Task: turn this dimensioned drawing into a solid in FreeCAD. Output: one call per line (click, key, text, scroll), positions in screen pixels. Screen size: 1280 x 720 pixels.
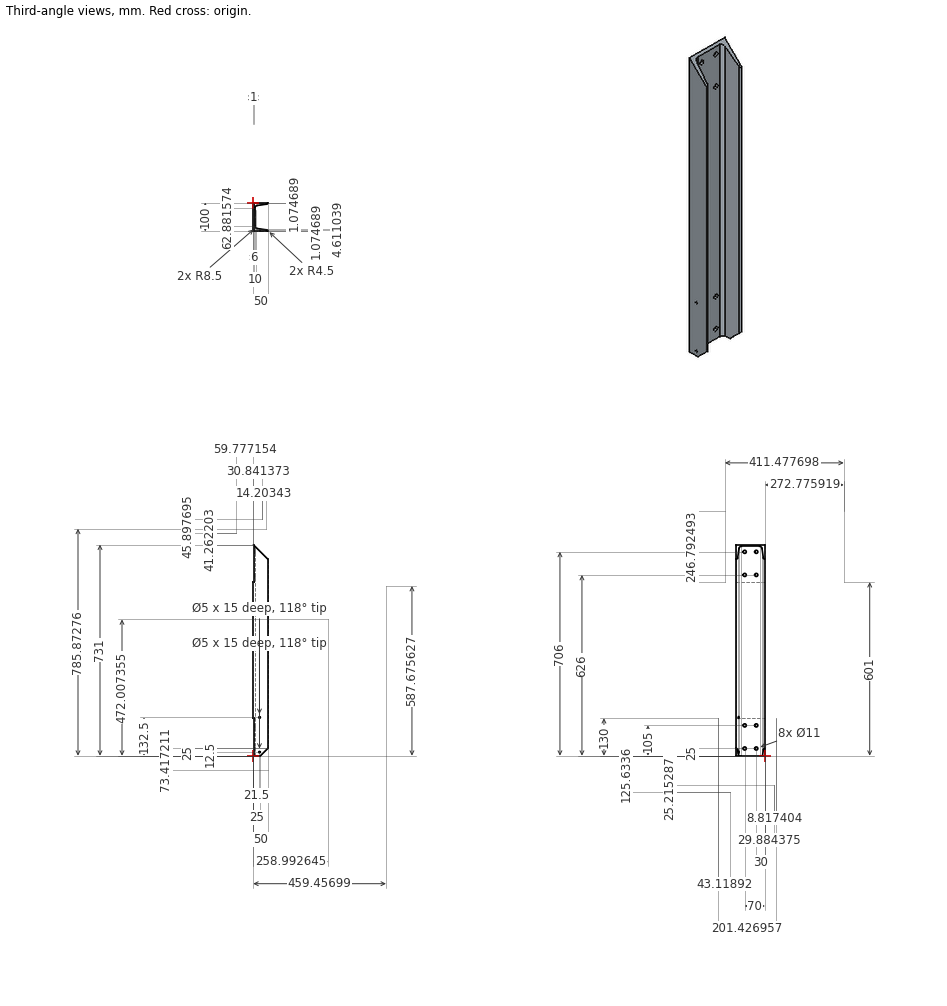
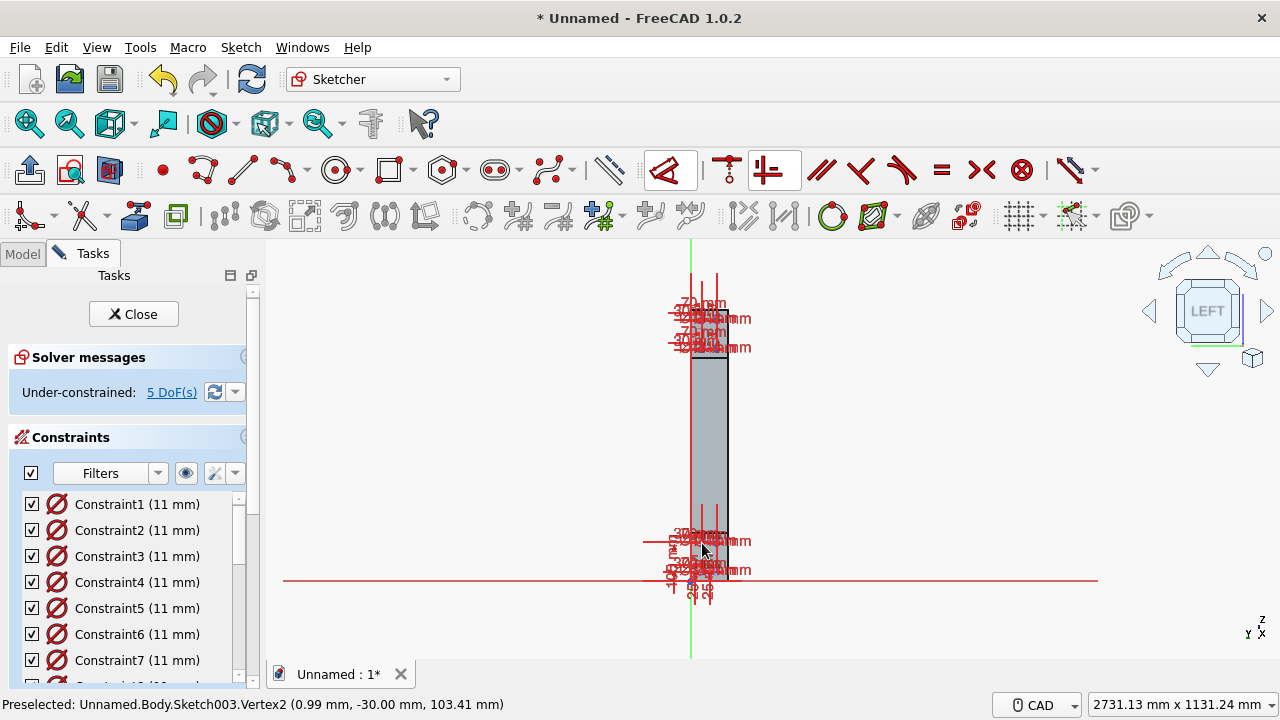
click(717, 543)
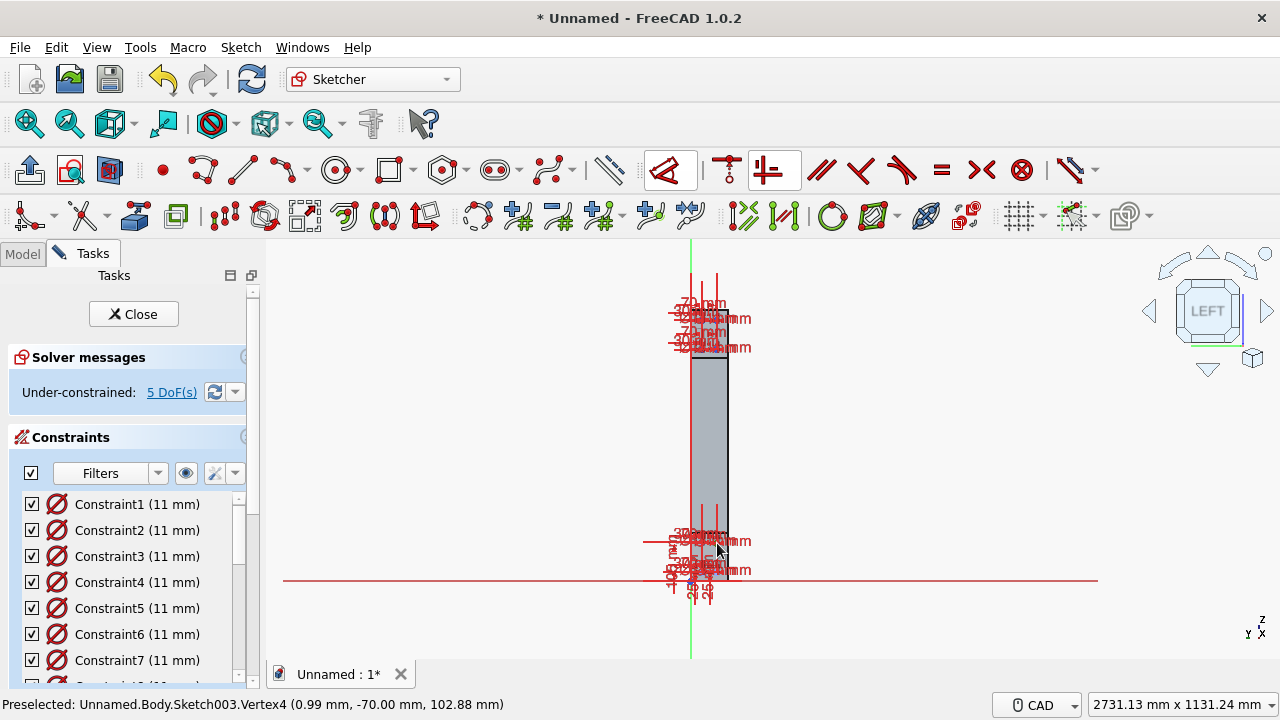
key(i)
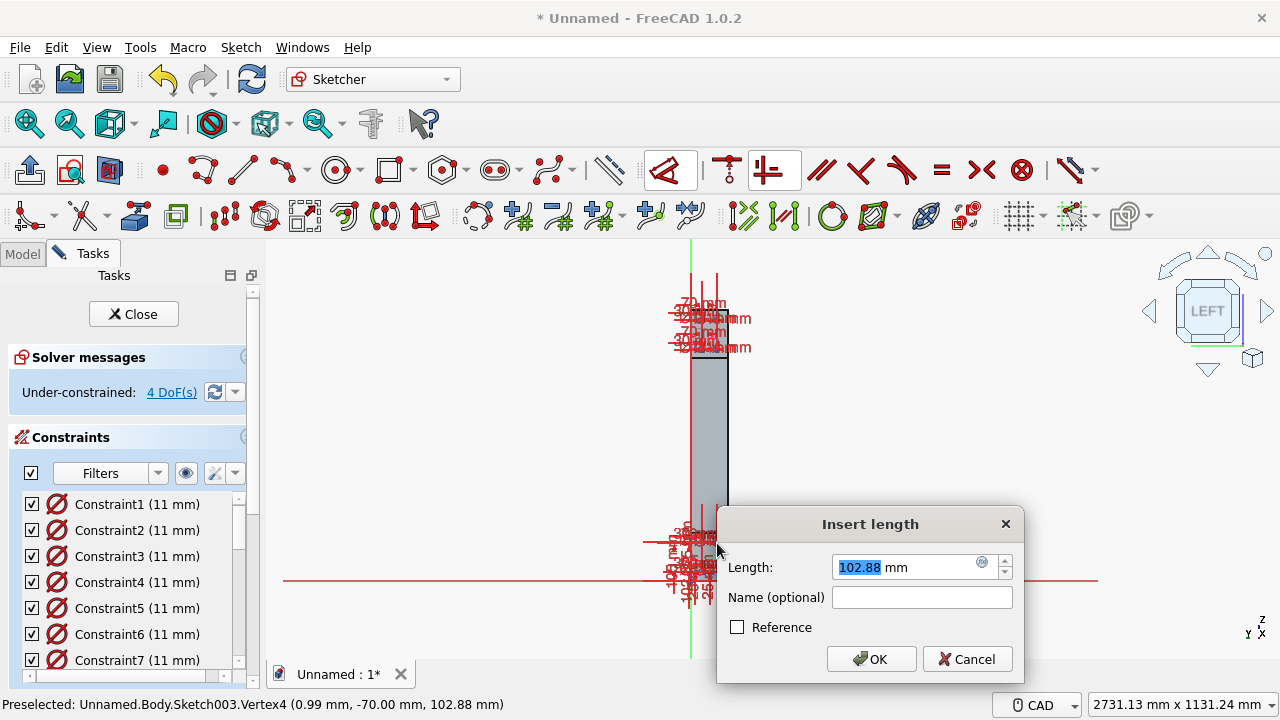
text(105)
key(Return)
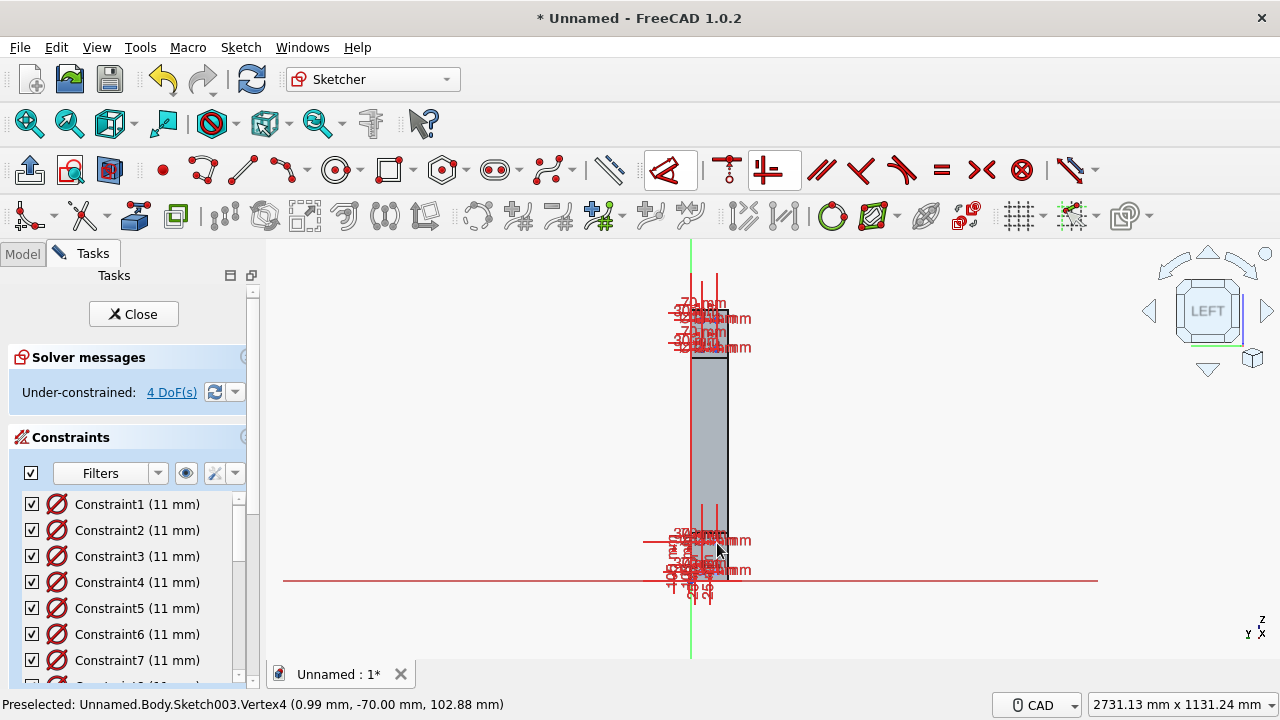
click(702, 350)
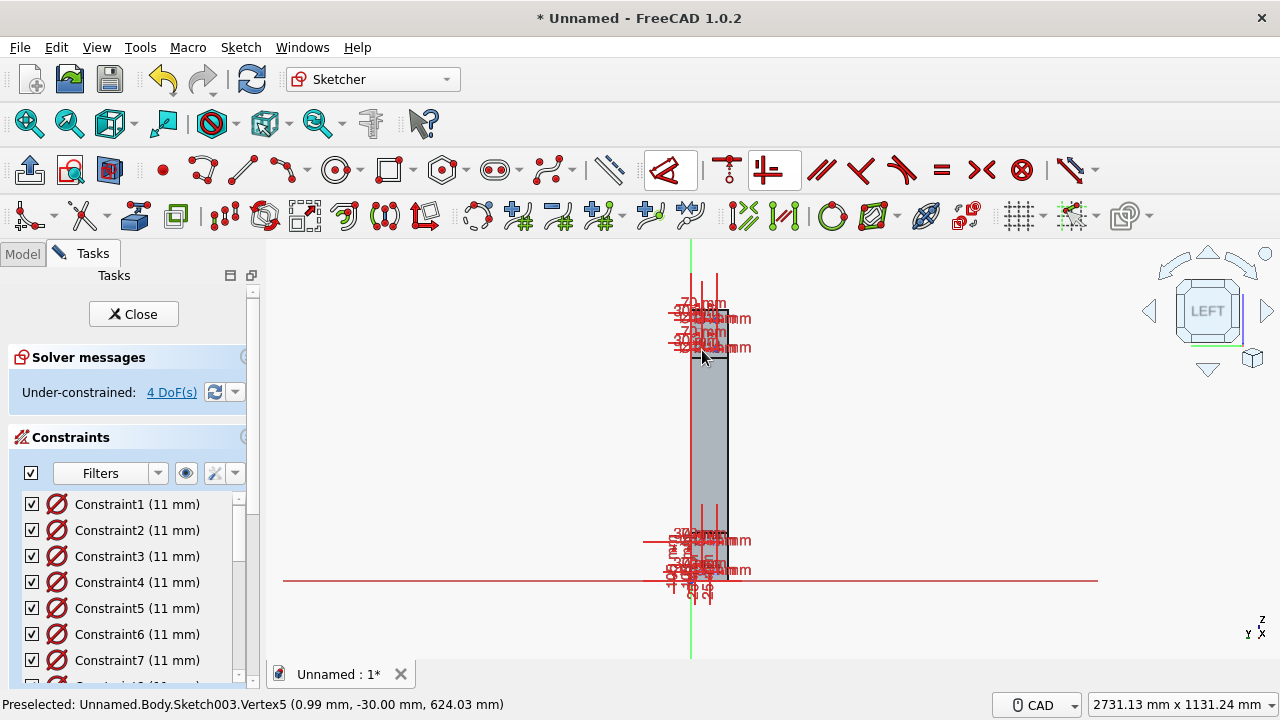
key(i)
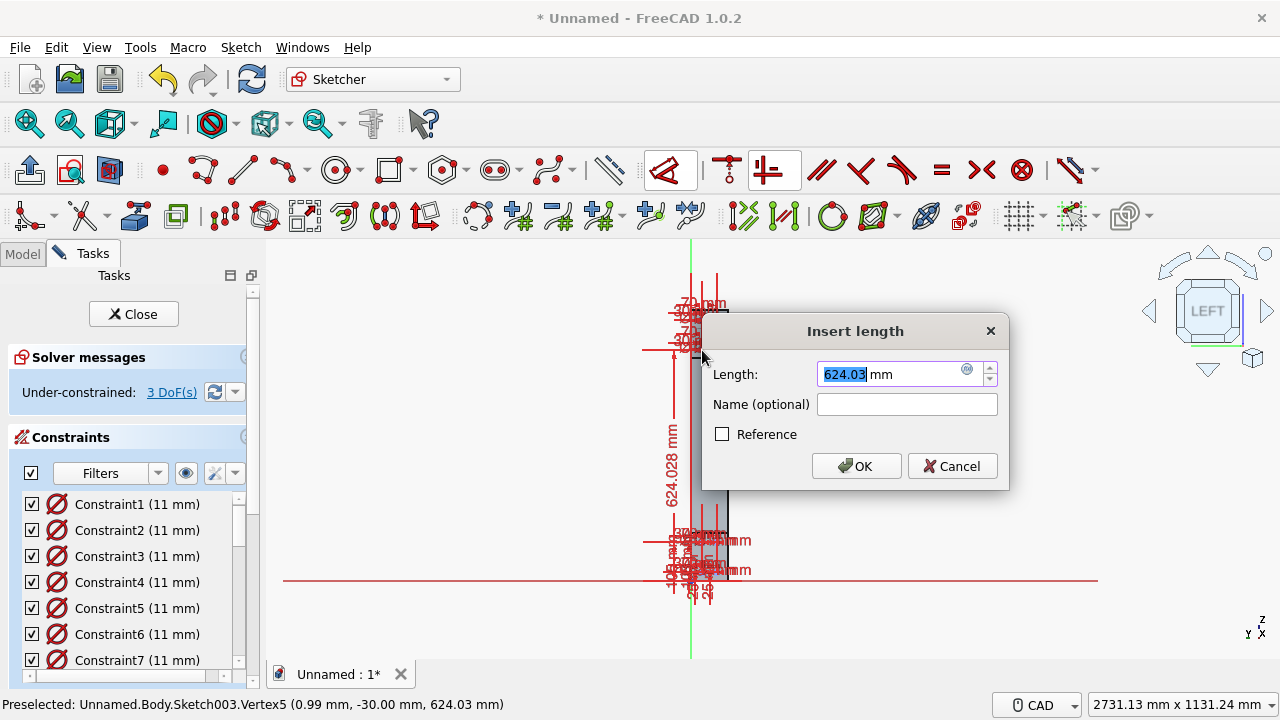
text(626)
key(Return)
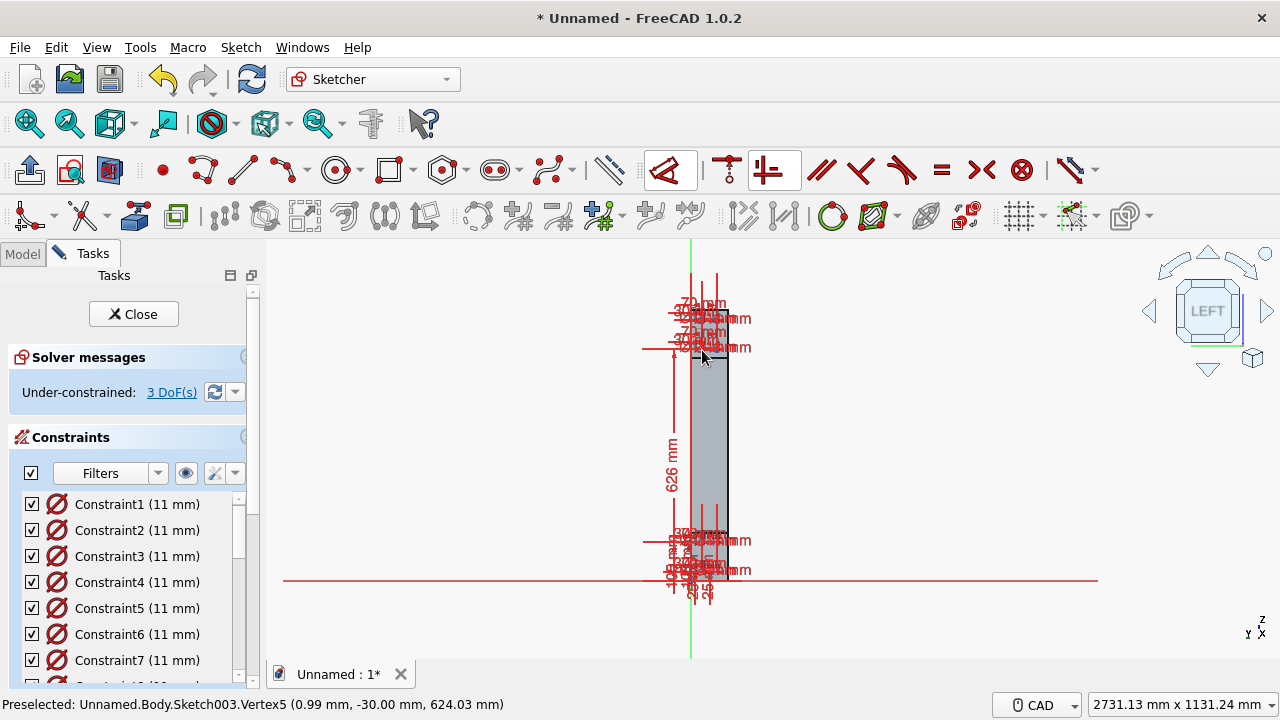
click(717, 321)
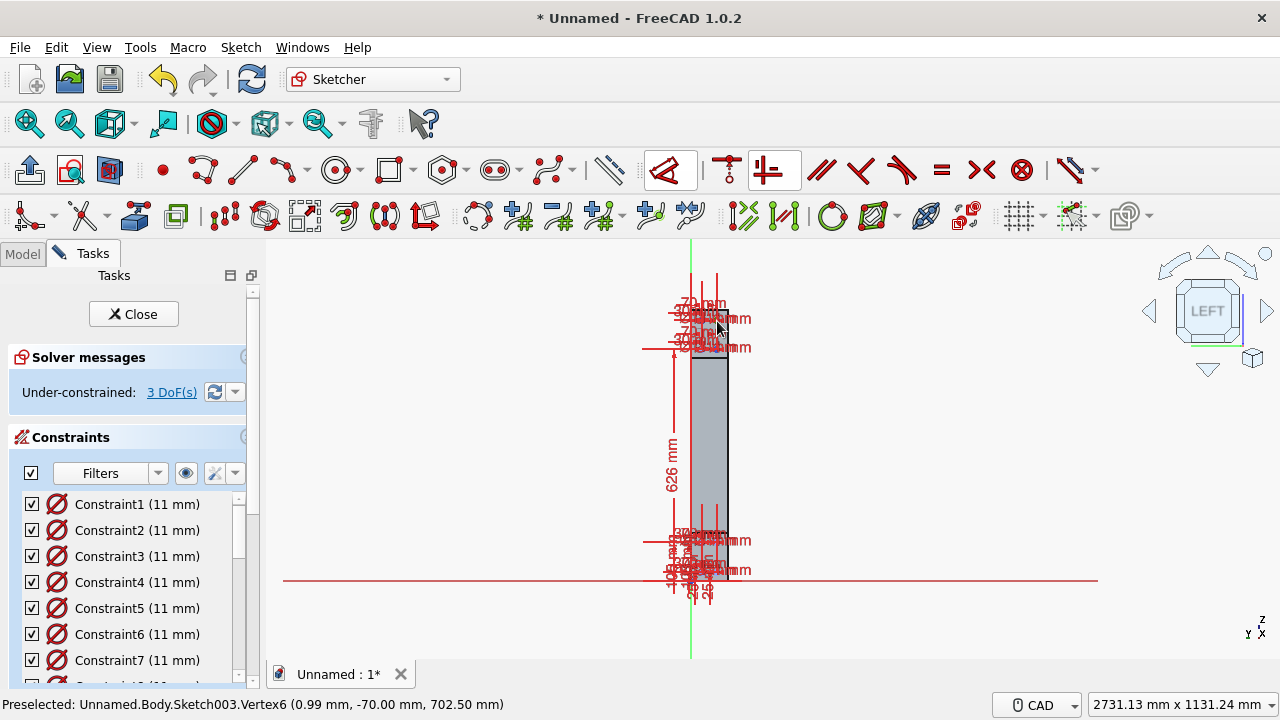
key(i)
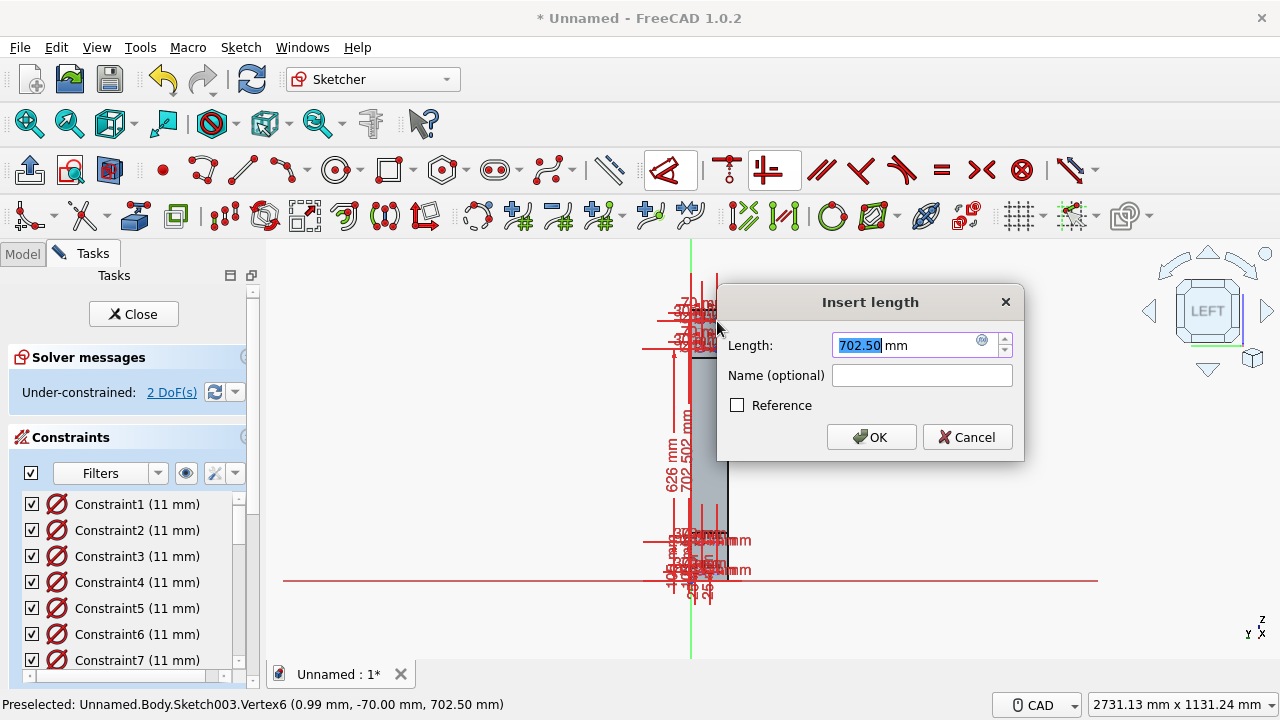
text(706)
key(Return)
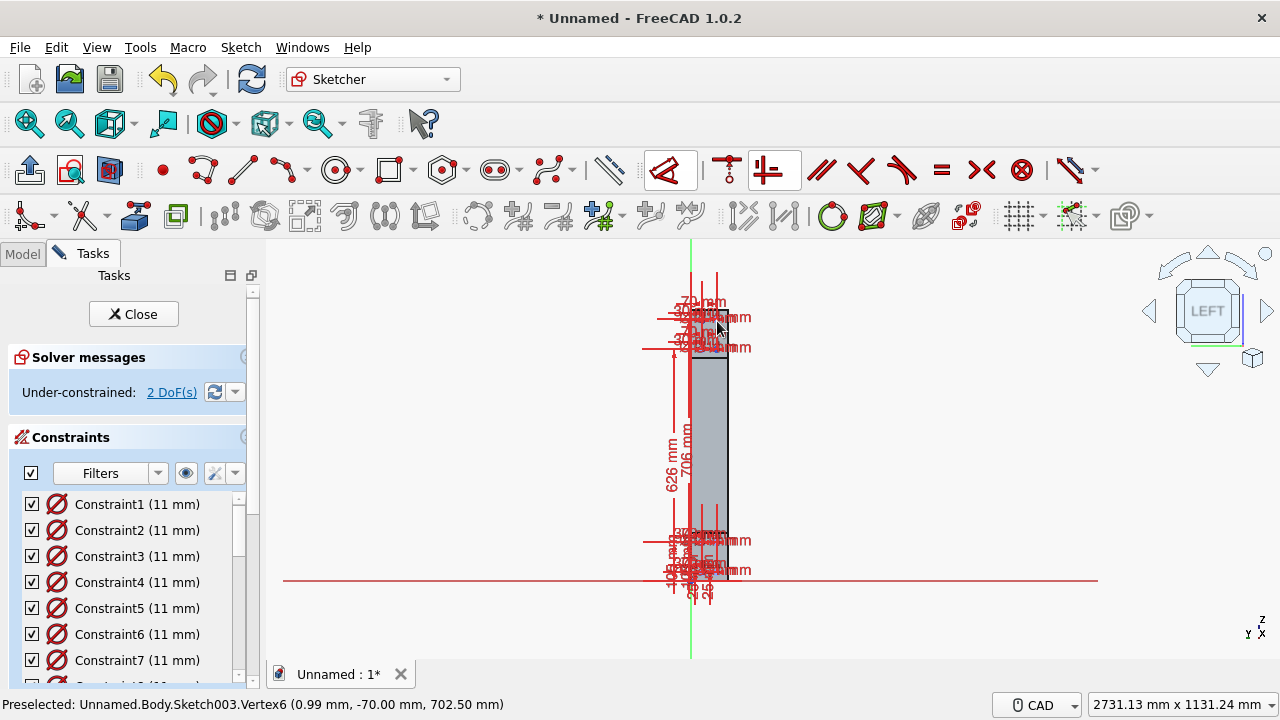
click(717, 349)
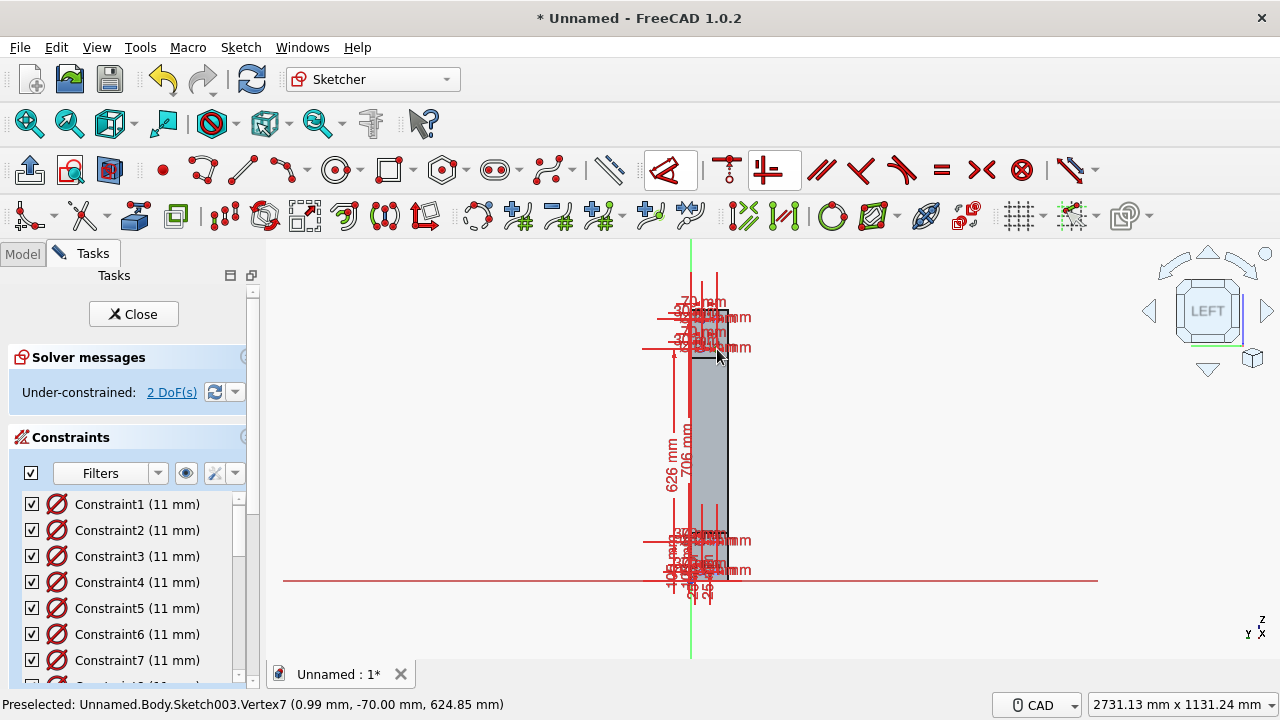
key(i)